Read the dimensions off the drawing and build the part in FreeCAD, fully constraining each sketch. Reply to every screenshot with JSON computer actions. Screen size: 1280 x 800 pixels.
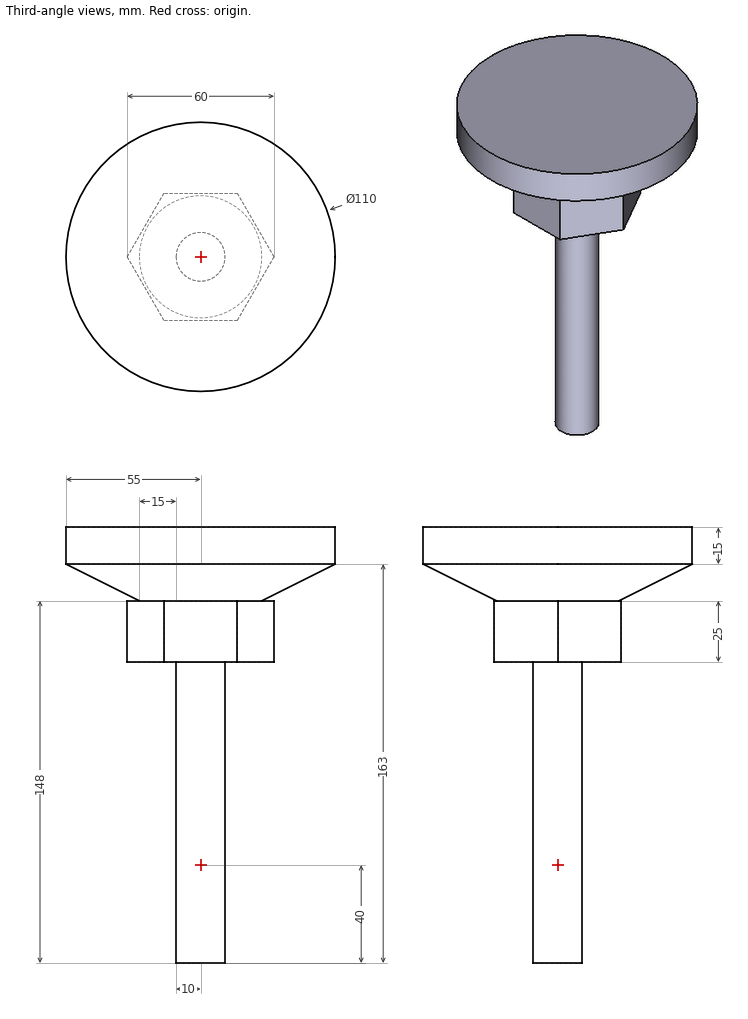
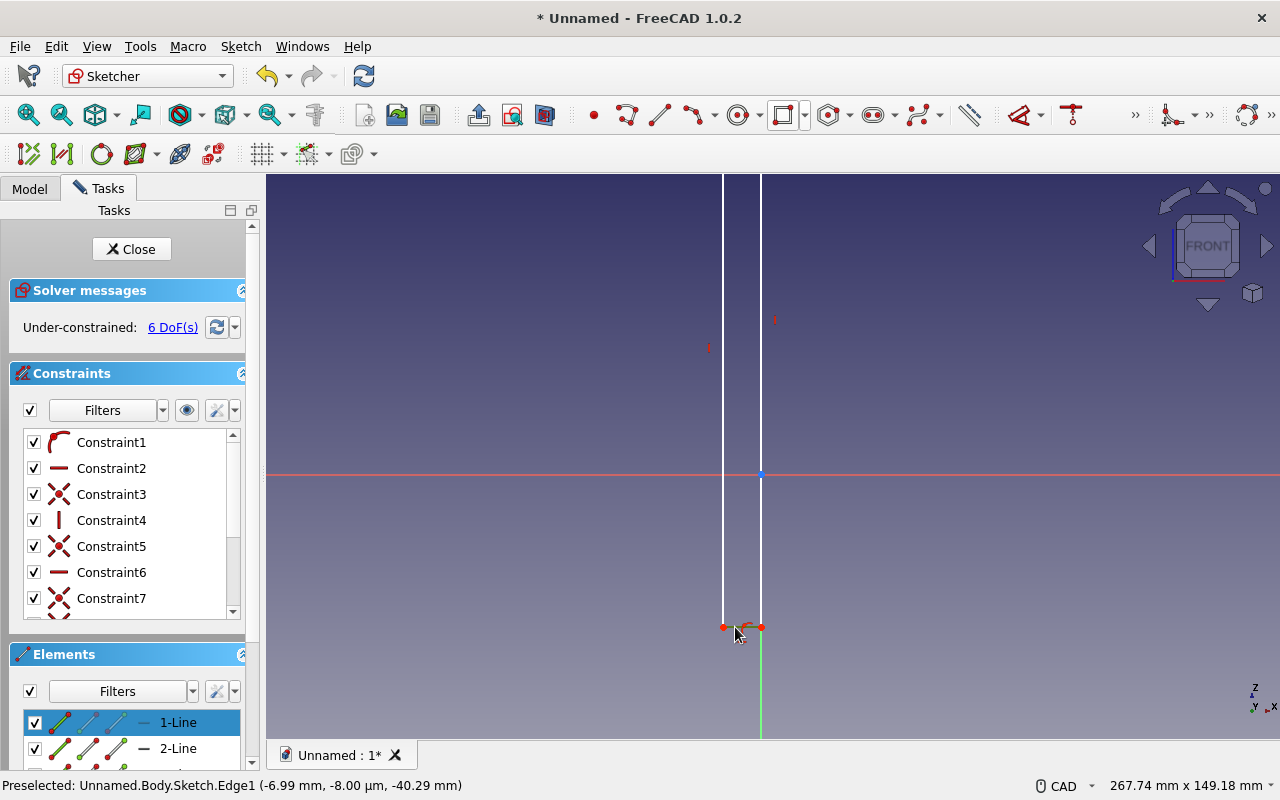
{"action": "left_click", "coordinate": [1040, 116]}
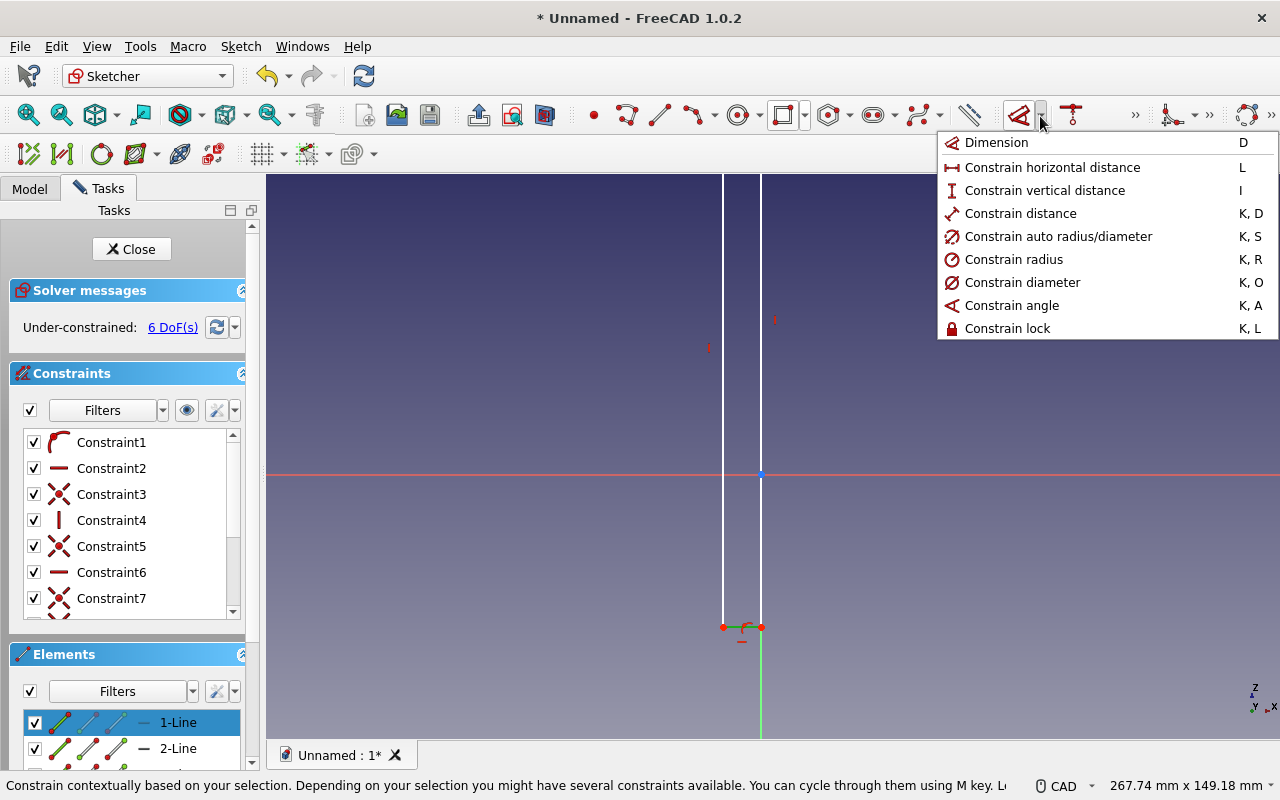
{"action": "left_click", "coordinate": [1108, 168]}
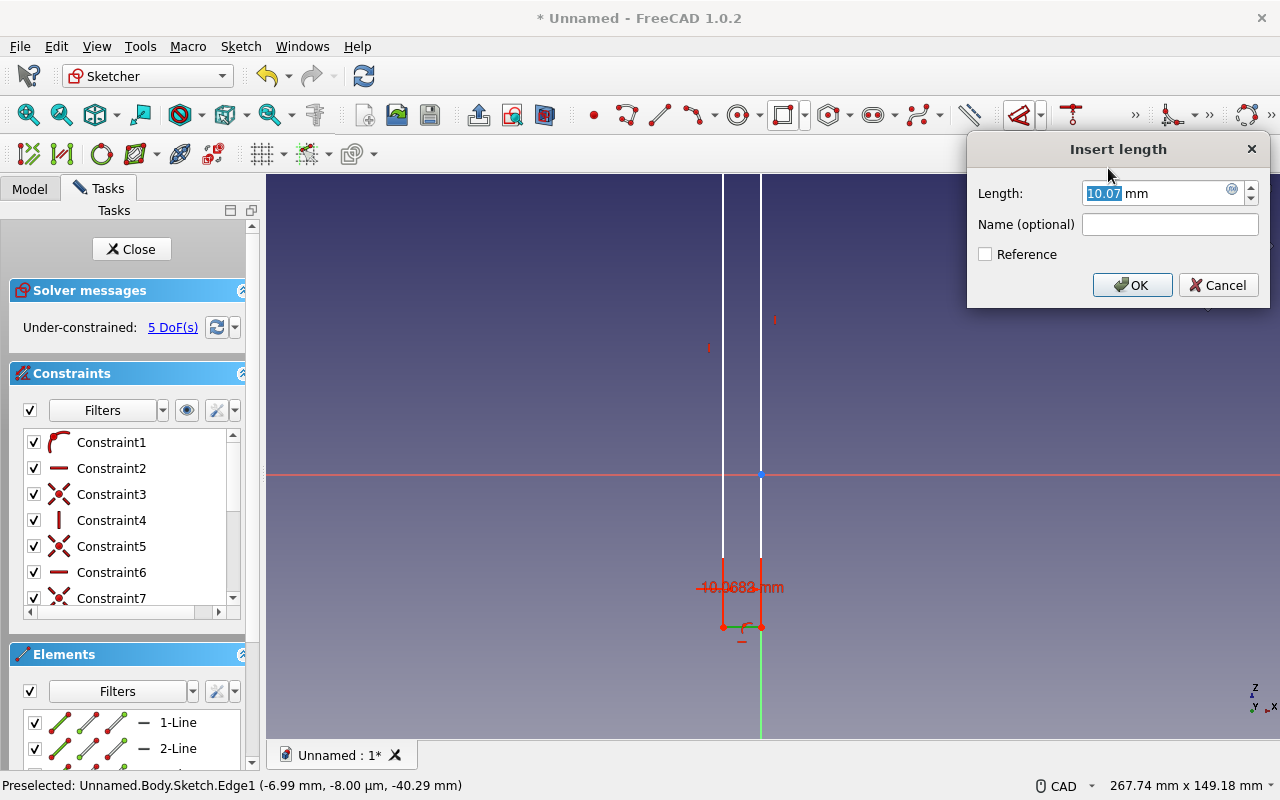
{"action": "type", "text": "10"}
{"action": "key", "text": "Return"}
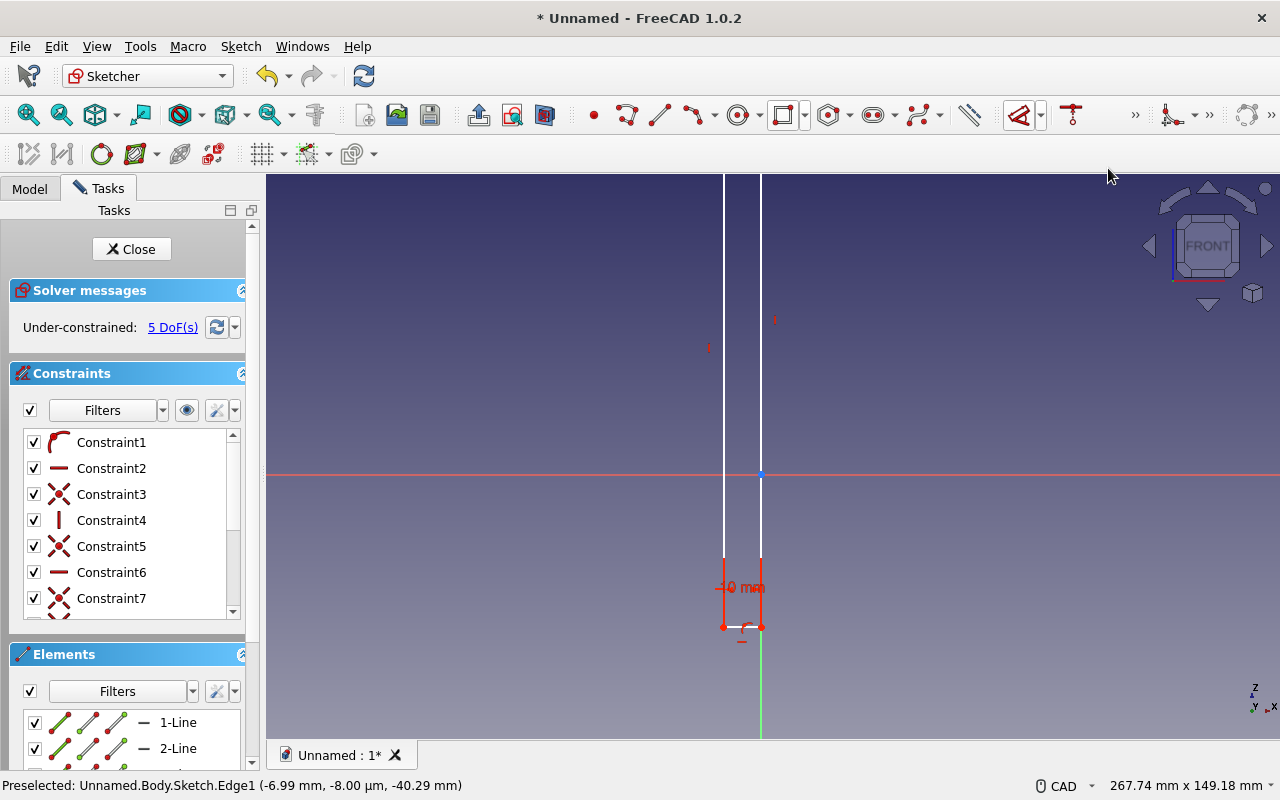
{"action": "scroll", "coordinate": [762, 626], "scroll_direction": "down", "scroll_amount": 3}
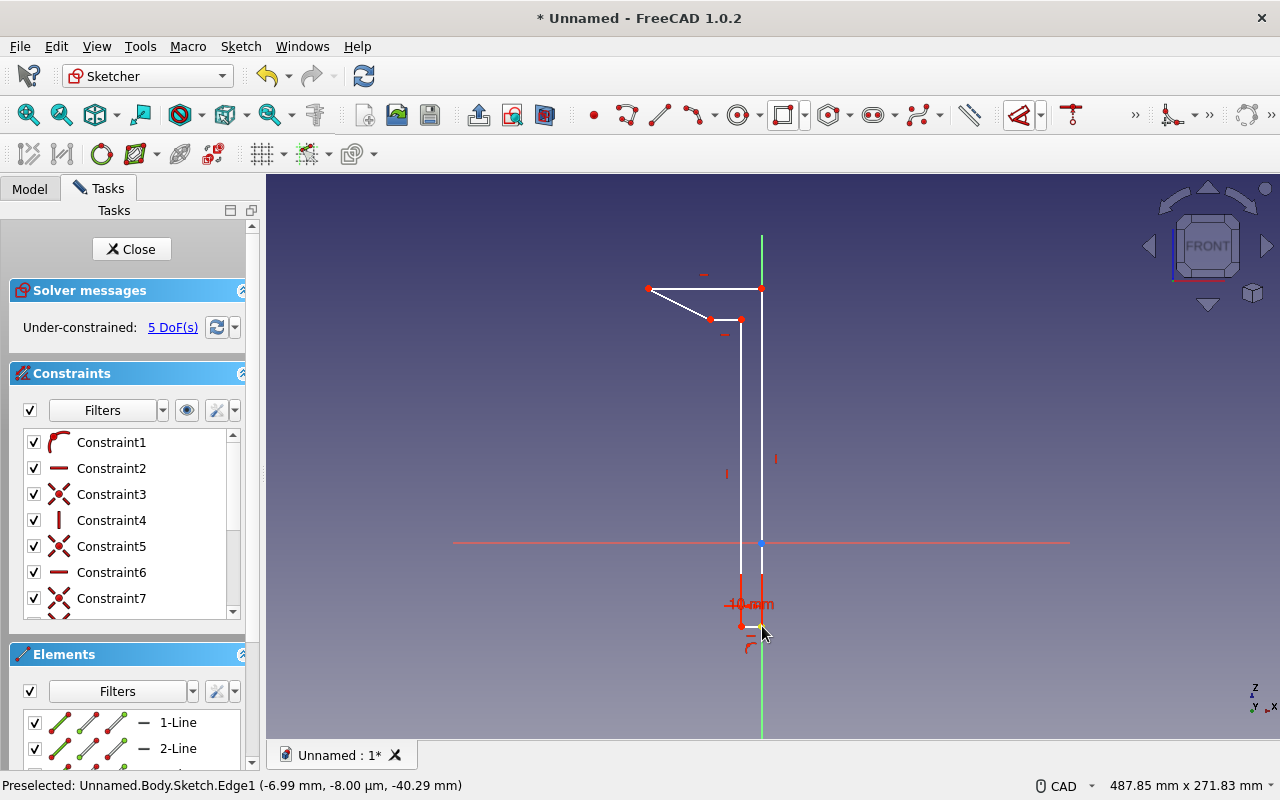
{"action": "scroll", "coordinate": [732, 320], "scroll_direction": "up", "scroll_amount": 2}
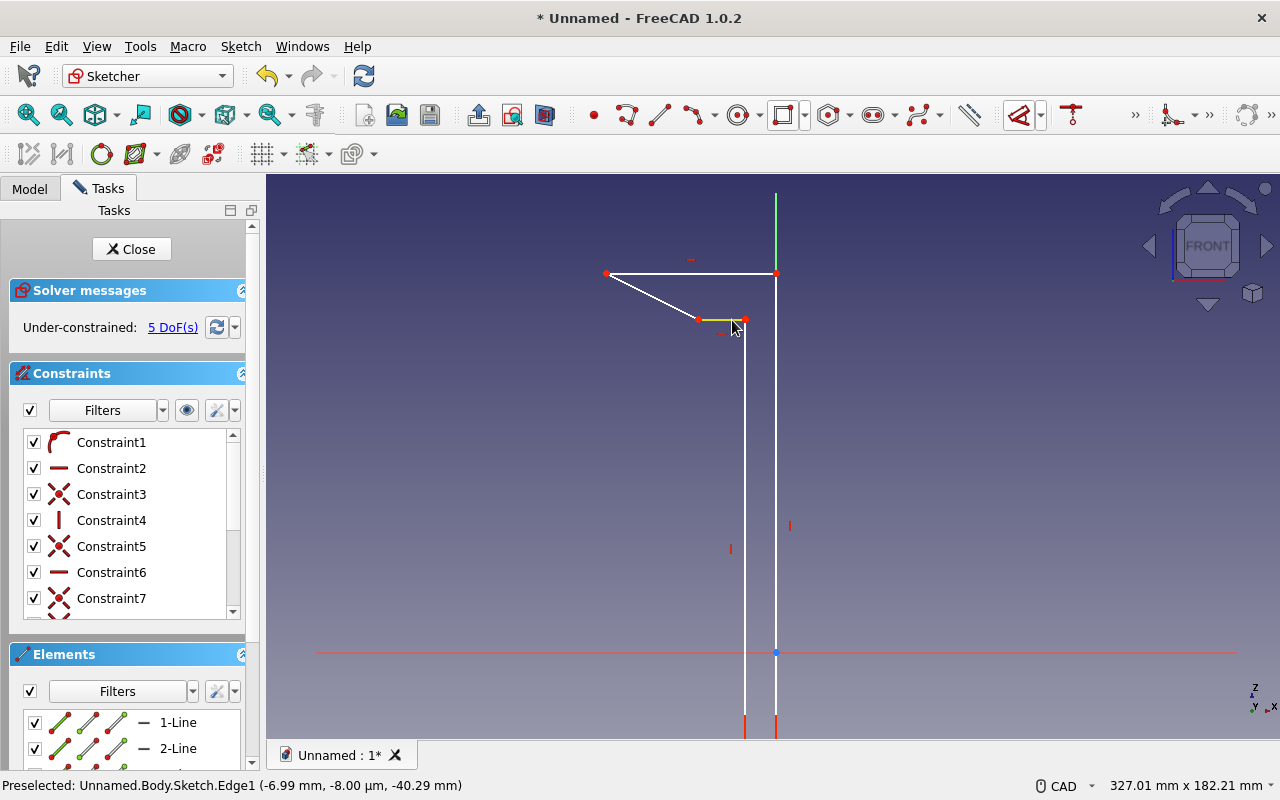
{"action": "left_click", "coordinate": [731, 320]}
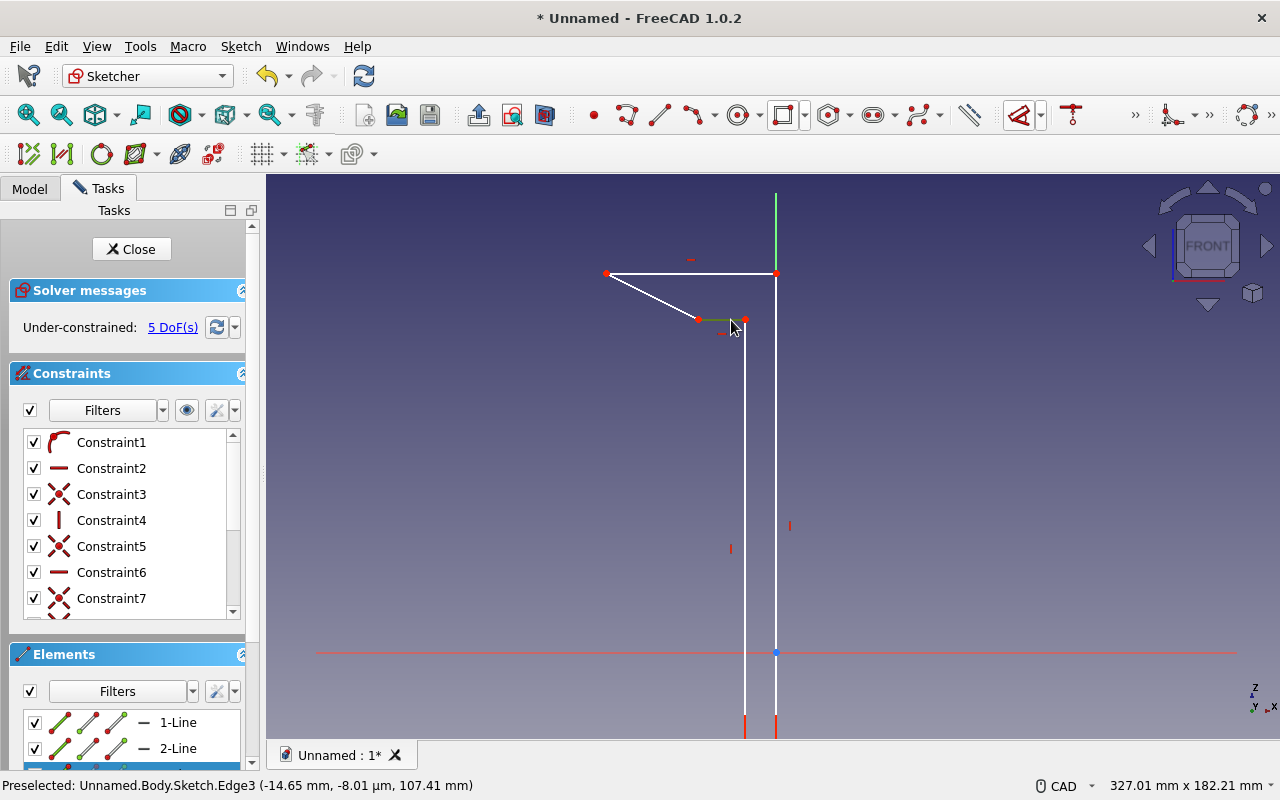
{"action": "left_click", "coordinate": [1040, 116]}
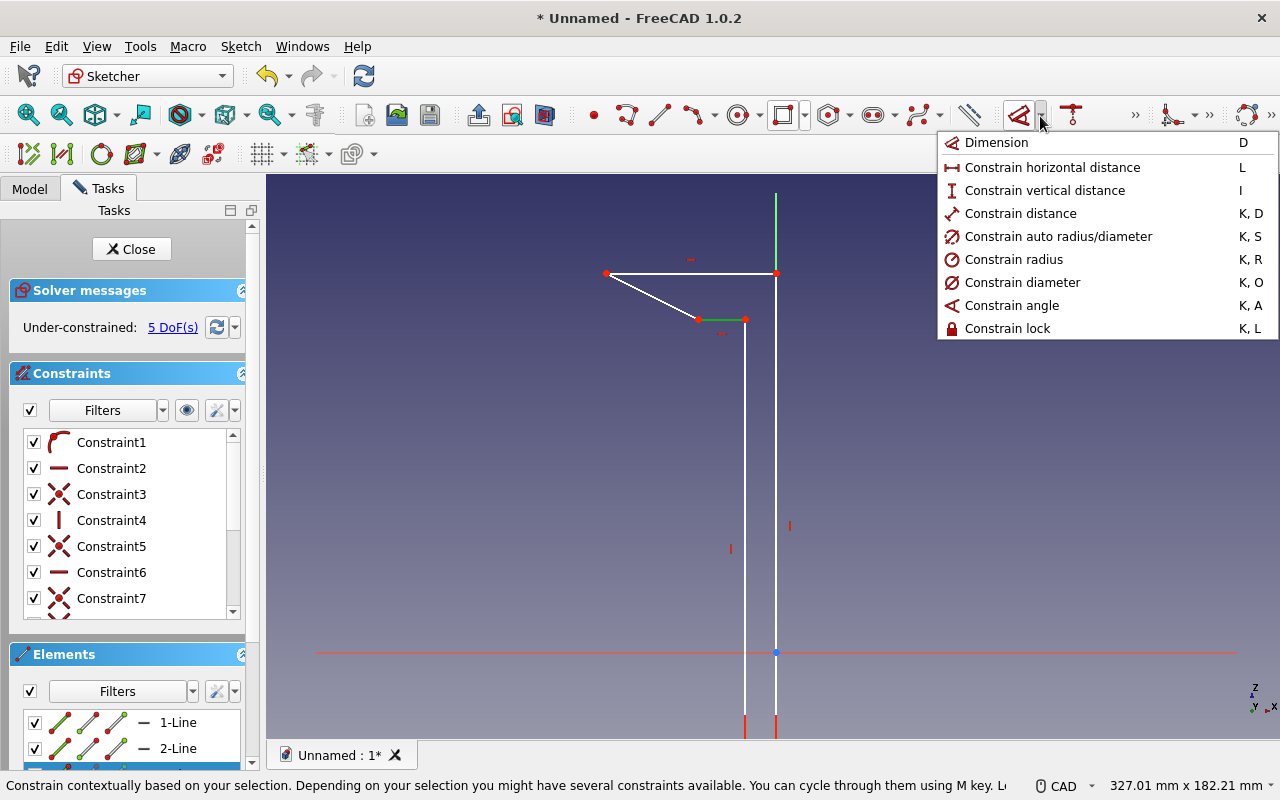
{"action": "left_click", "coordinate": [1108, 168]}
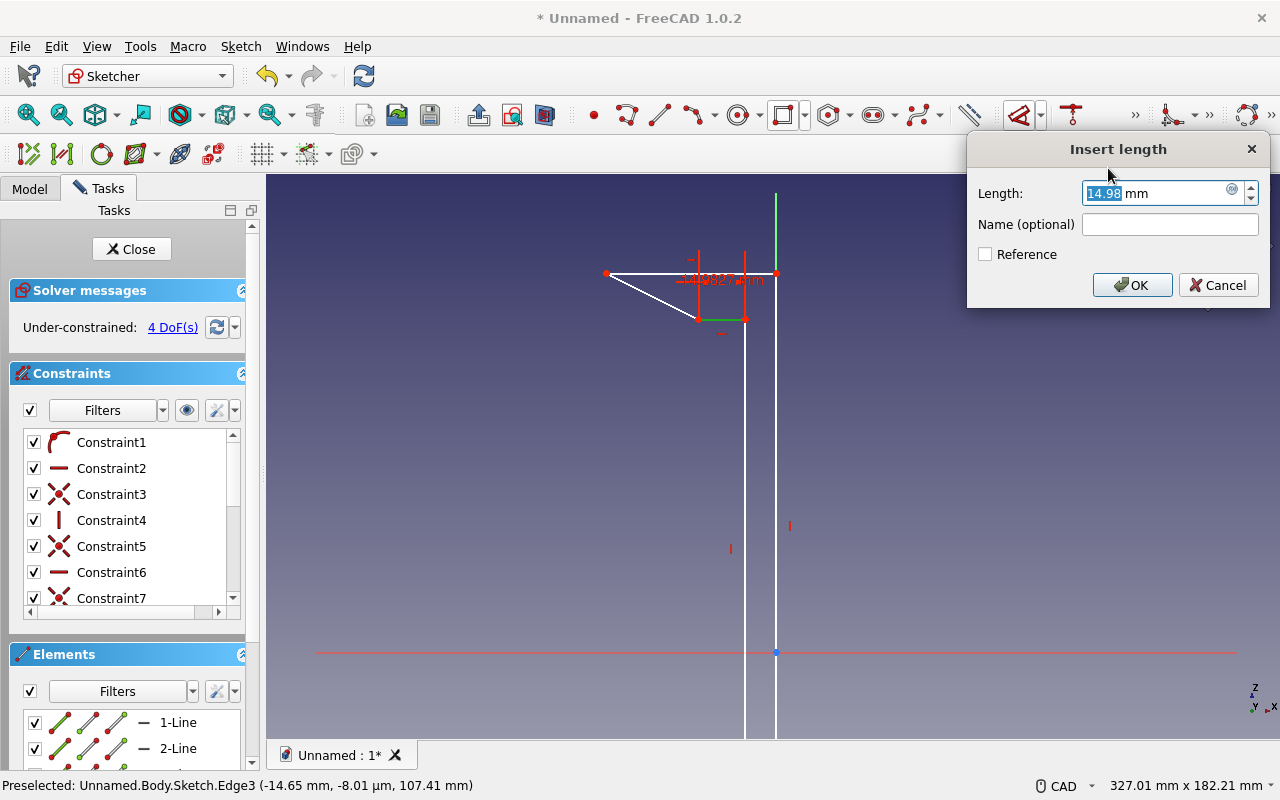
{"action": "type", "text": "15"}
{"action": "key", "text": "Return"}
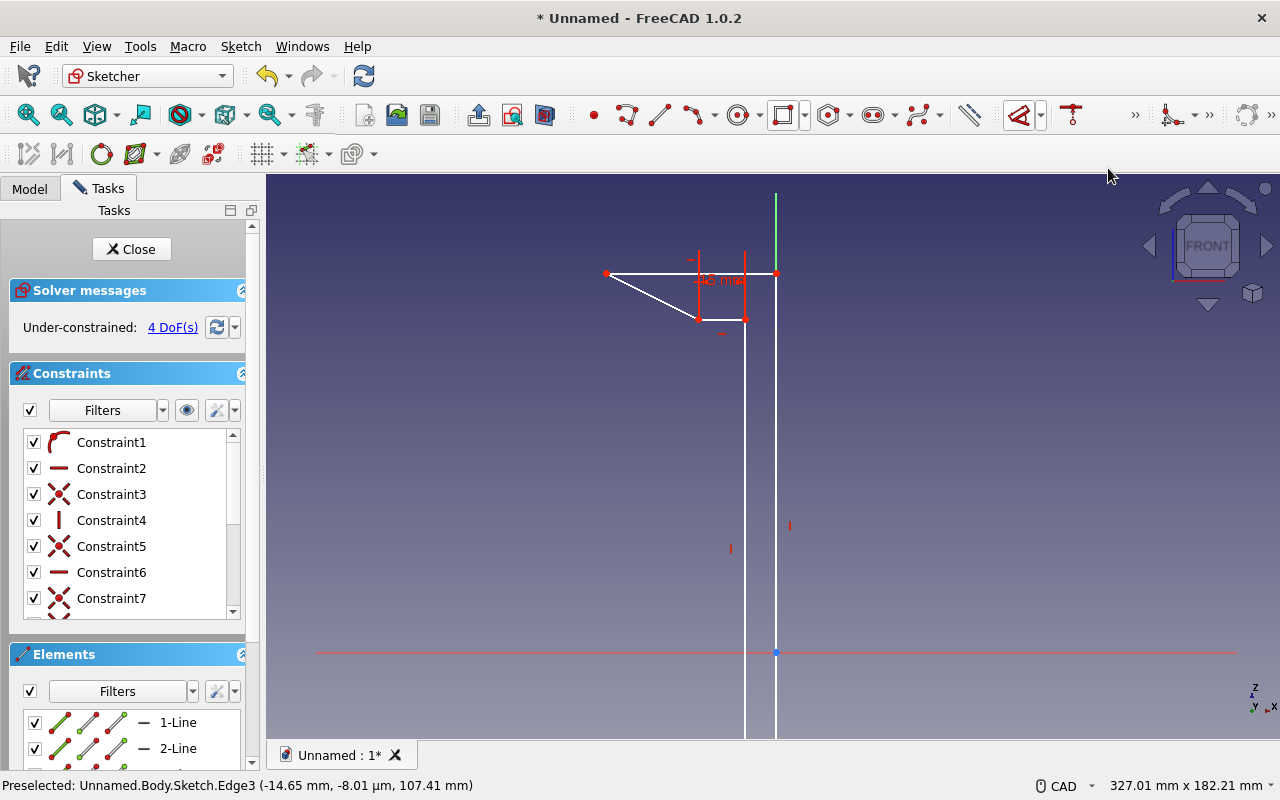
{"action": "left_click", "coordinate": [657, 274]}